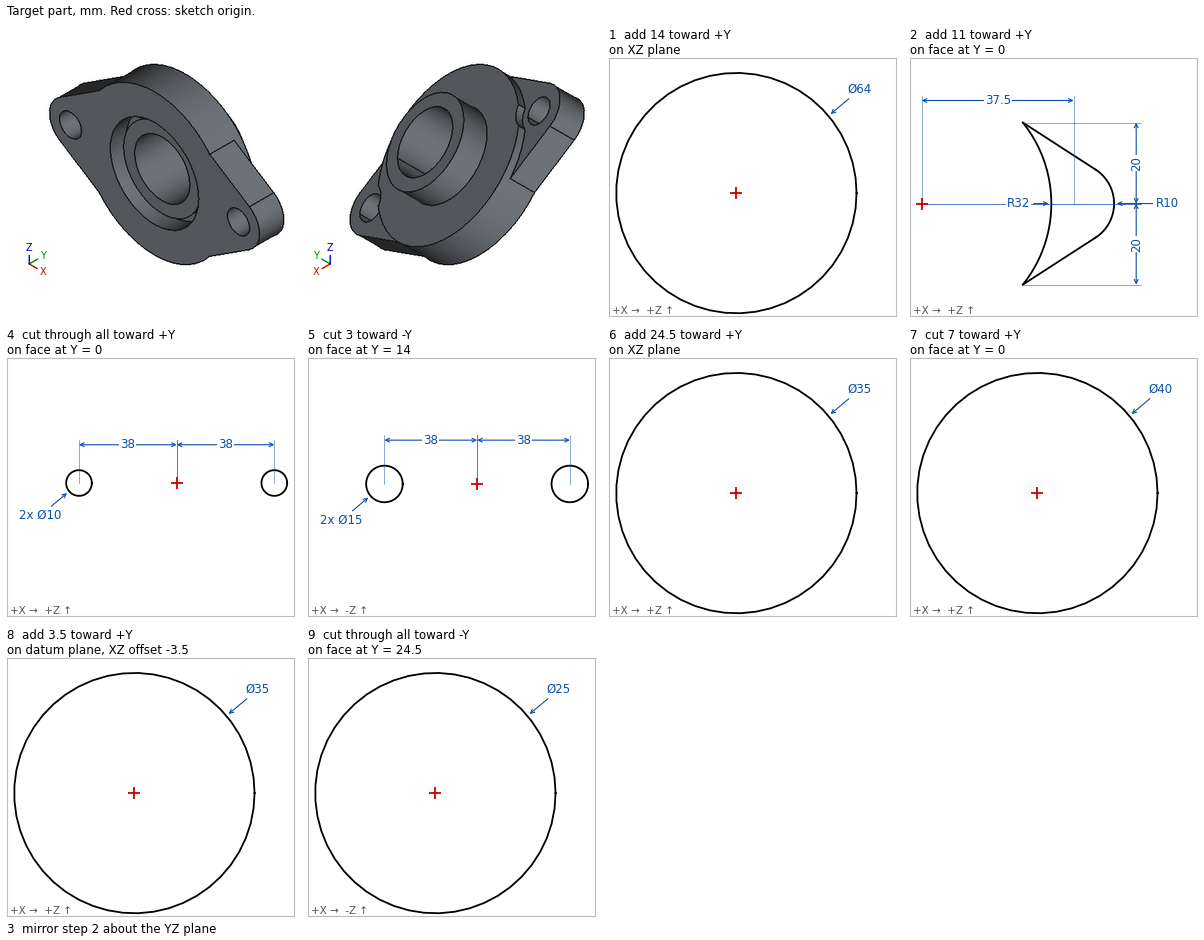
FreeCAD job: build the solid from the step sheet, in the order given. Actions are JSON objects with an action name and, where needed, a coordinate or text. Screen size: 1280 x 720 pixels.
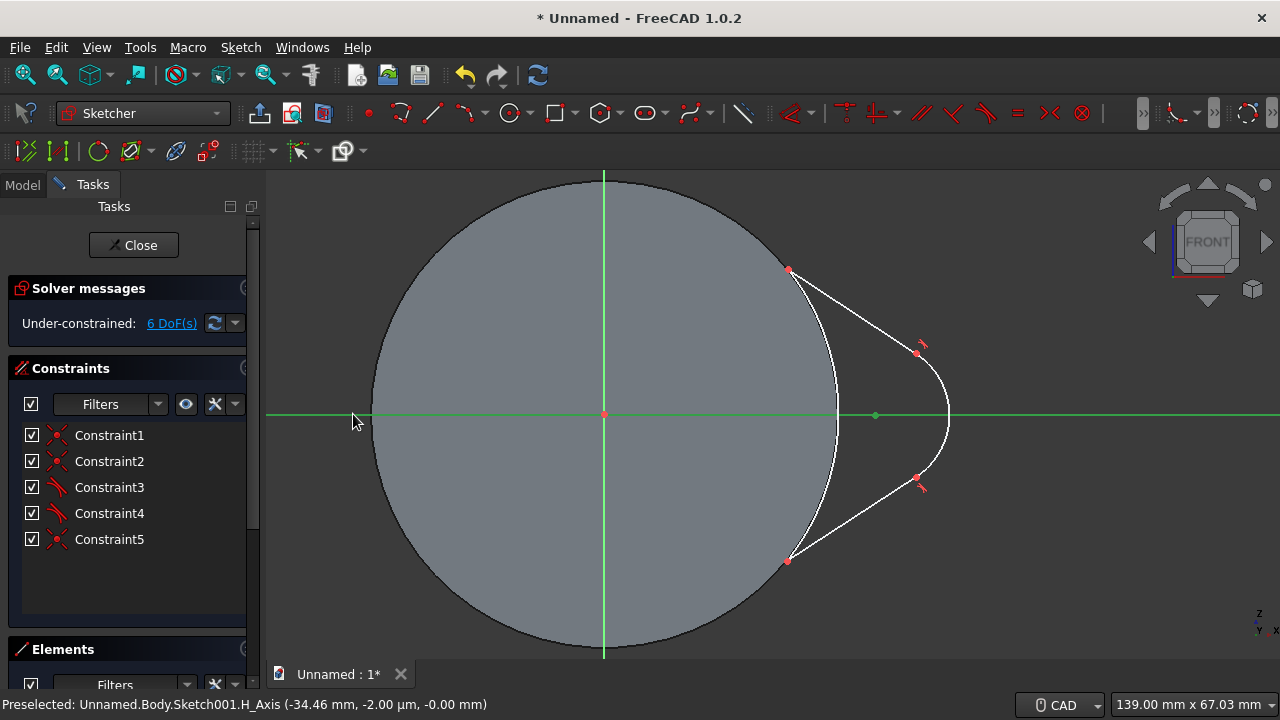
{"action": "left_click", "coordinate": [846, 114]}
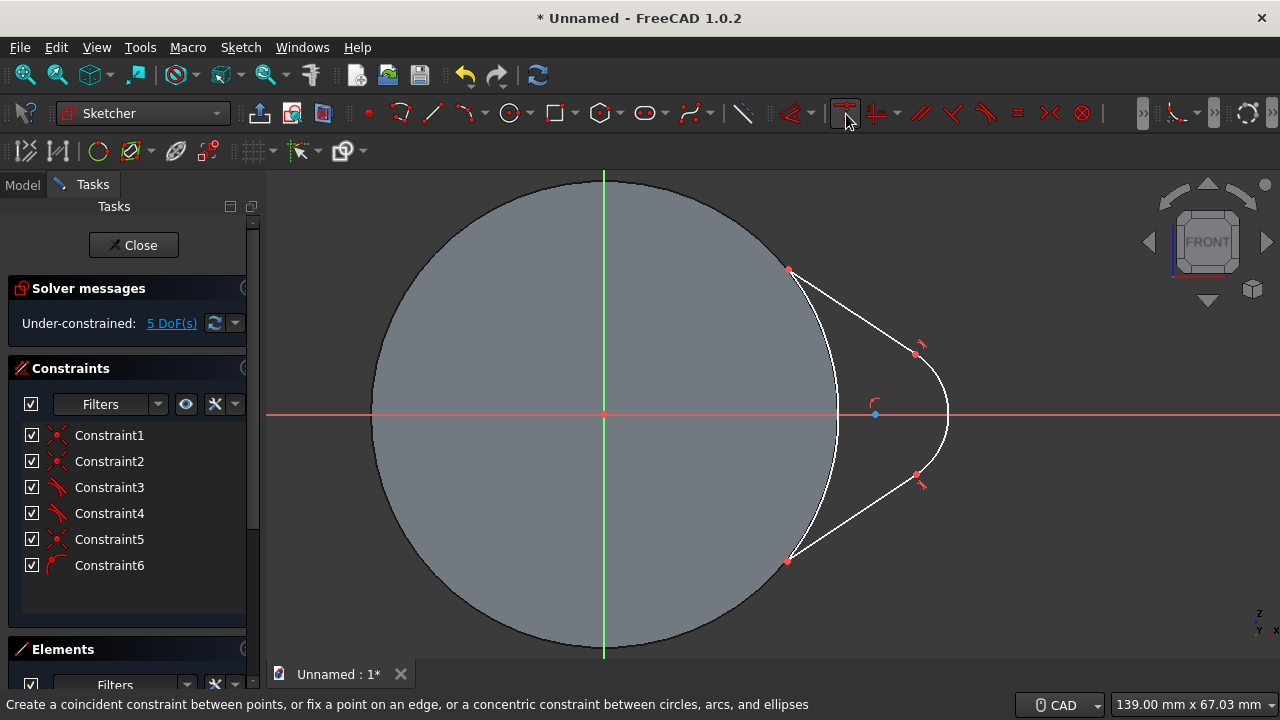
{"action": "left_click", "coordinate": [790, 114]}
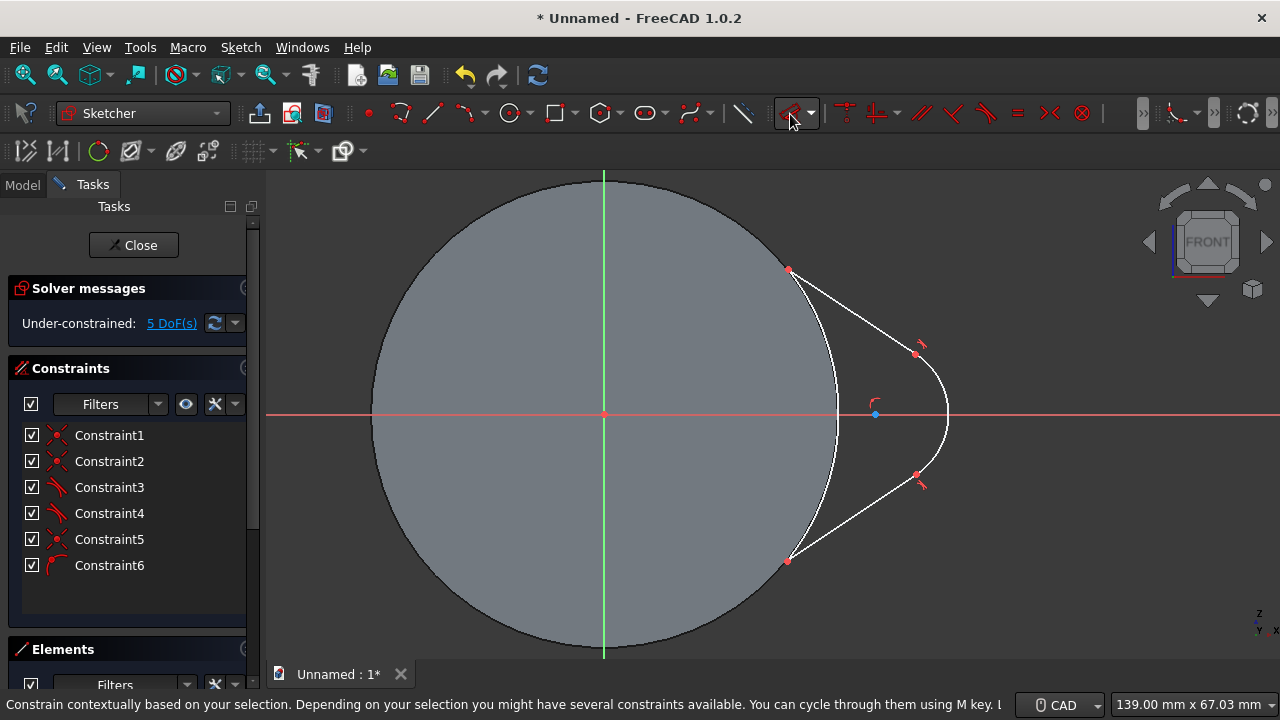
{"action": "left_click", "coordinate": [830, 478]}
{"action": "left_click", "coordinate": [861, 487]}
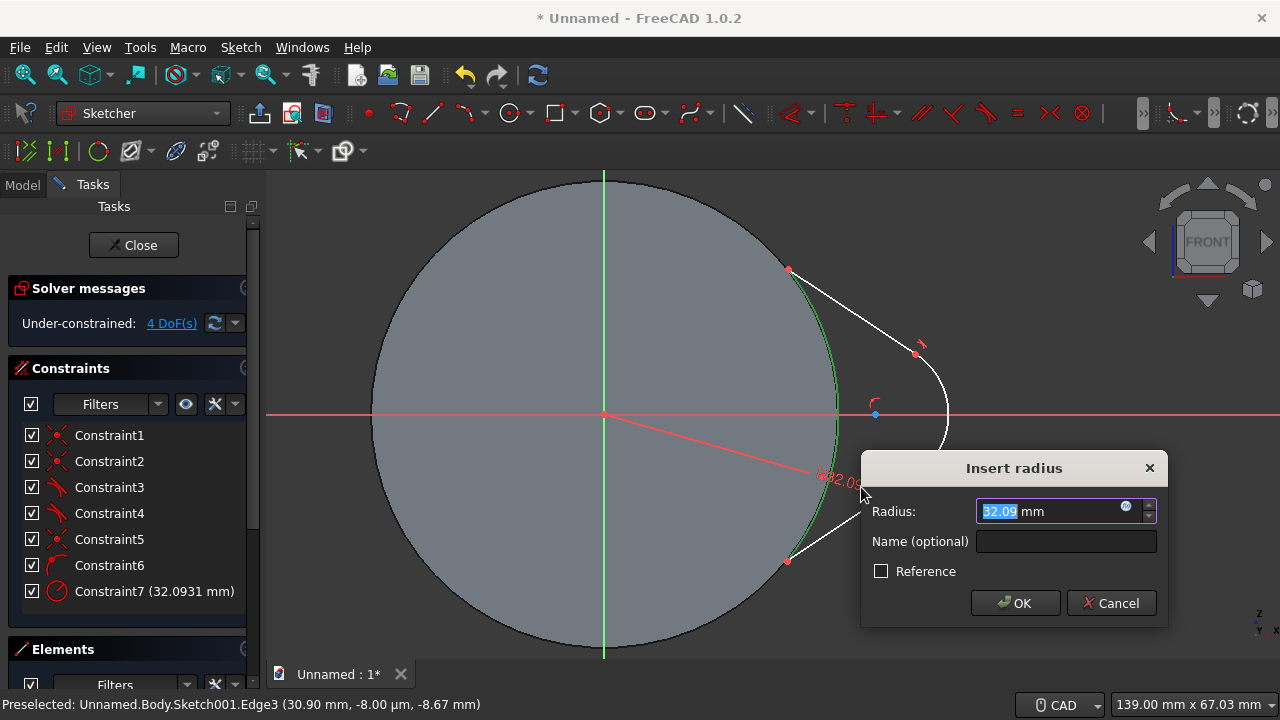
{"action": "type", "text": "32"}
{"action": "key", "text": "Return"}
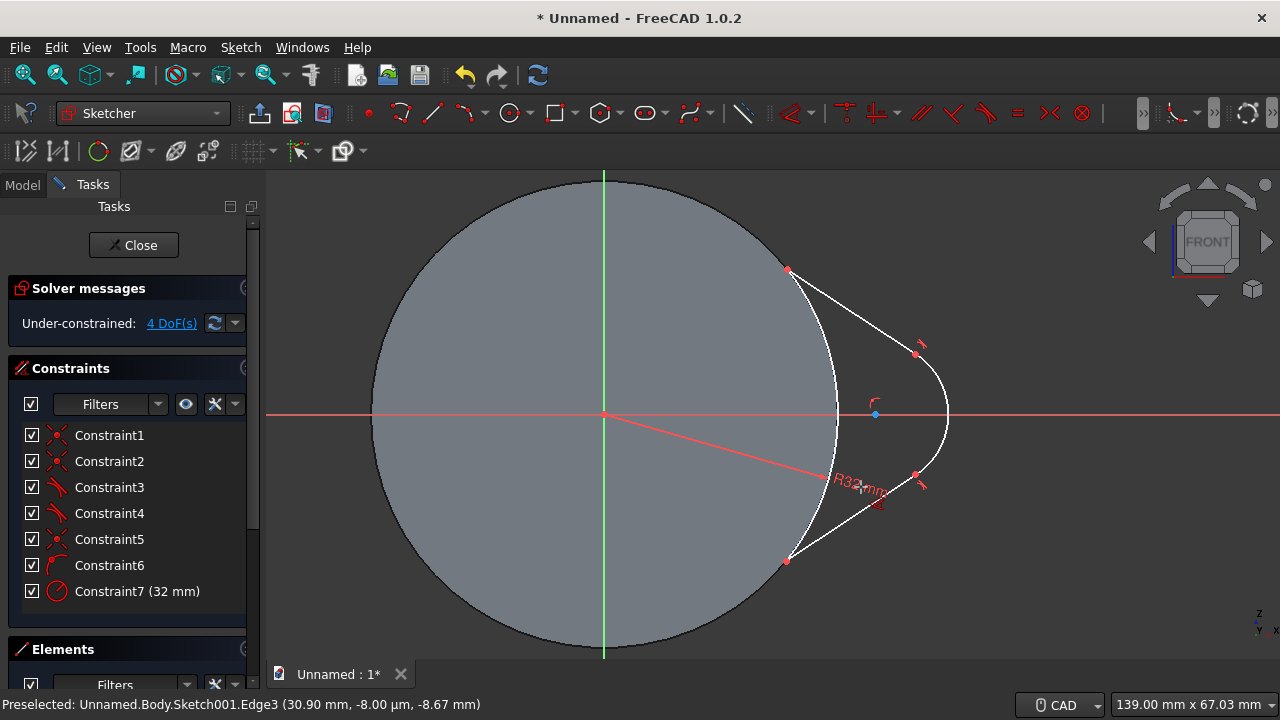
{"action": "left_click", "coordinate": [943, 442]}
{"action": "left_click", "coordinate": [973, 454]}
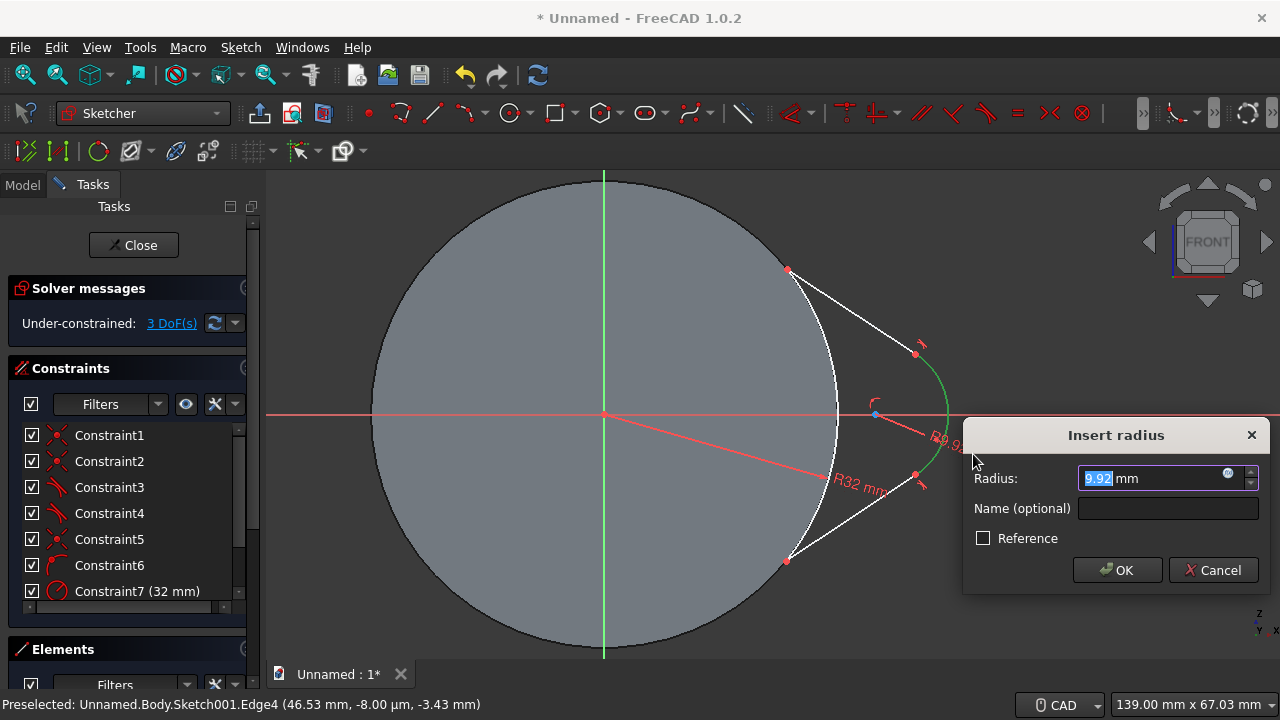
{"action": "type", "text": "10"}
{"action": "key", "text": "Return"}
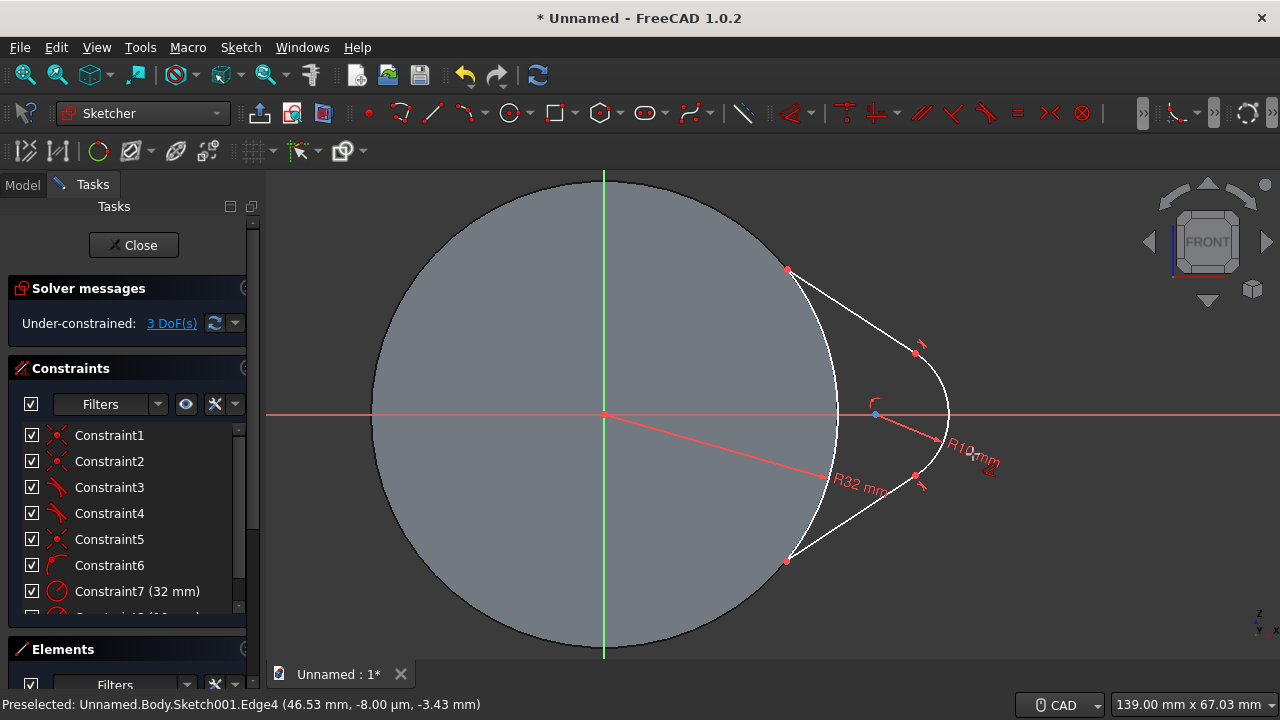
{"action": "left_click", "coordinate": [786, 561]}
{"action": "left_click", "coordinate": [570, 488]}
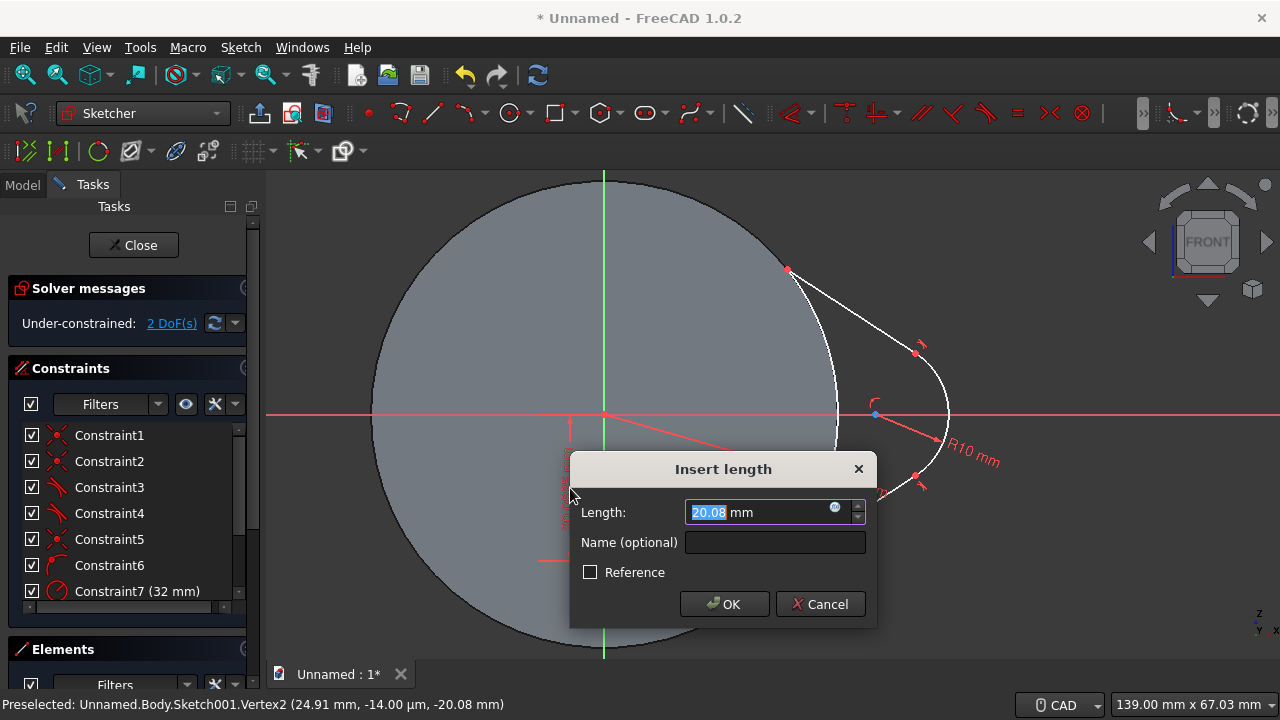
{"action": "type", "text": "20"}
{"action": "key", "text": "Return"}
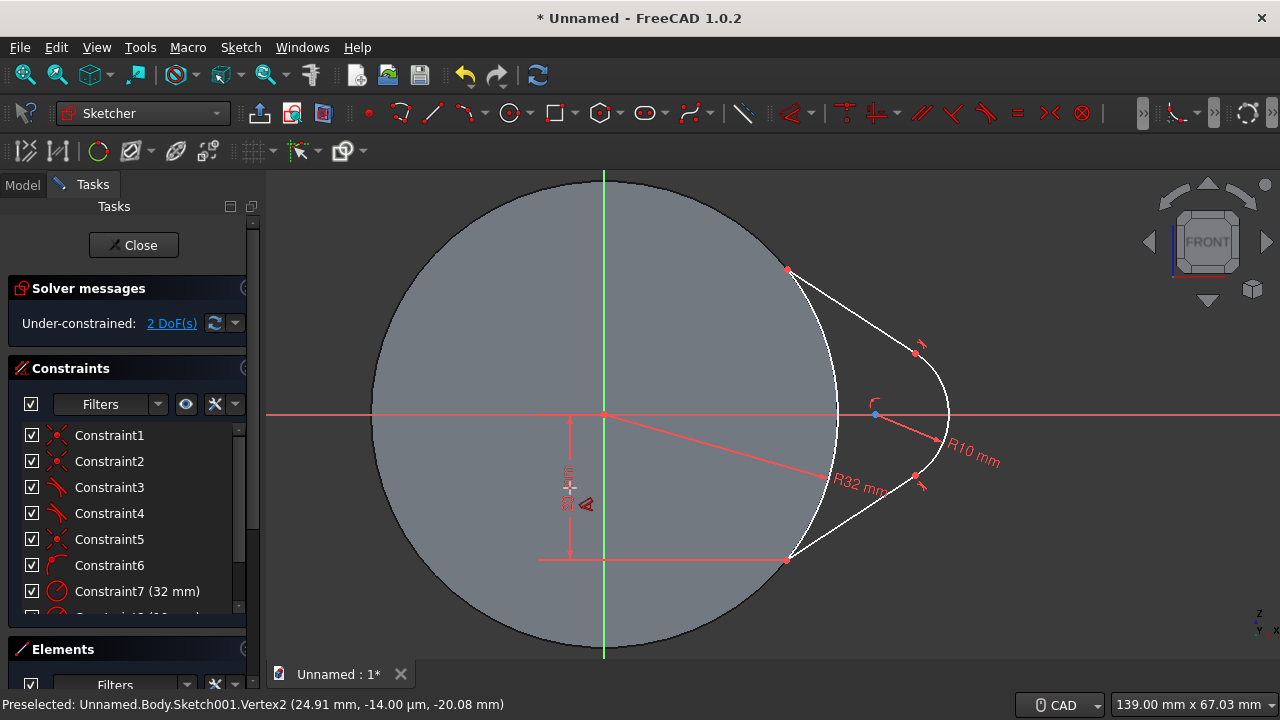
{"action": "left_click", "coordinate": [788, 270]}
{"action": "left_click", "coordinate": [570, 342]}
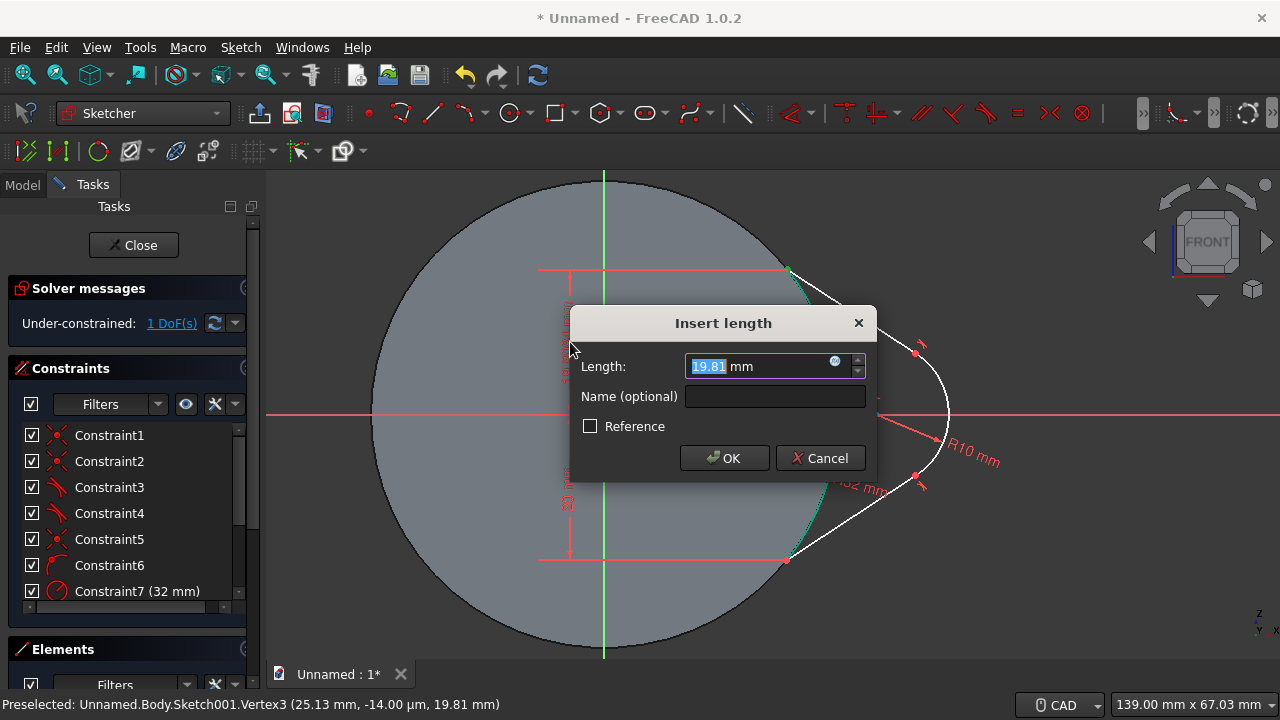
{"action": "type", "text": "20"}
{"action": "key", "text": "Return"}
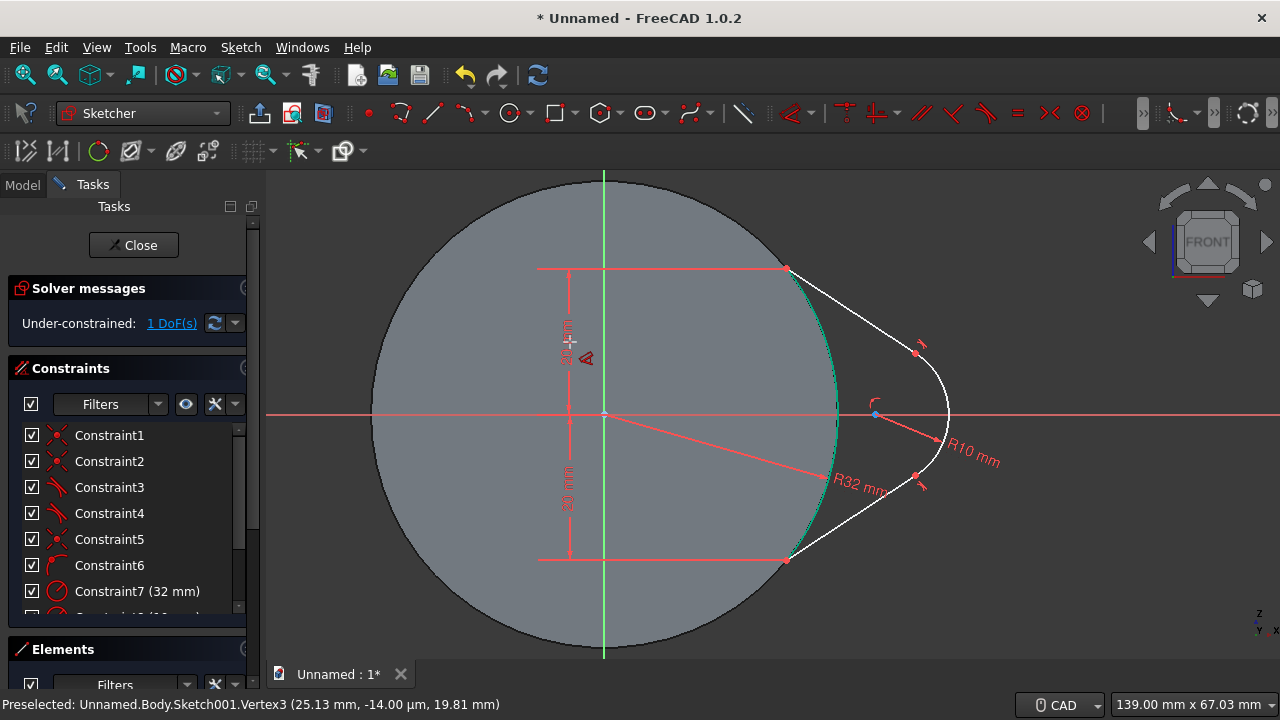
{"action": "left_click", "coordinate": [876, 414]}
{"action": "left_click", "coordinate": [740, 448]}